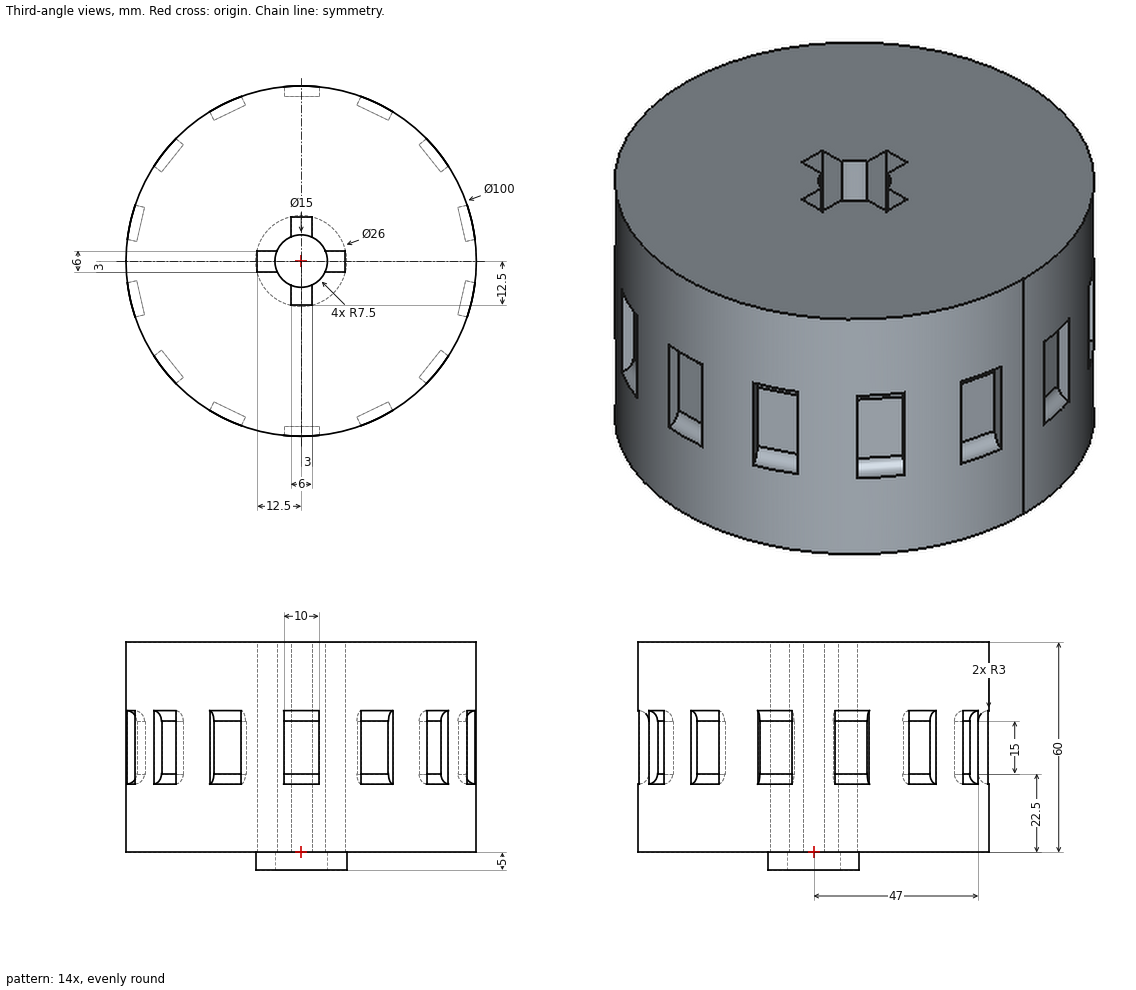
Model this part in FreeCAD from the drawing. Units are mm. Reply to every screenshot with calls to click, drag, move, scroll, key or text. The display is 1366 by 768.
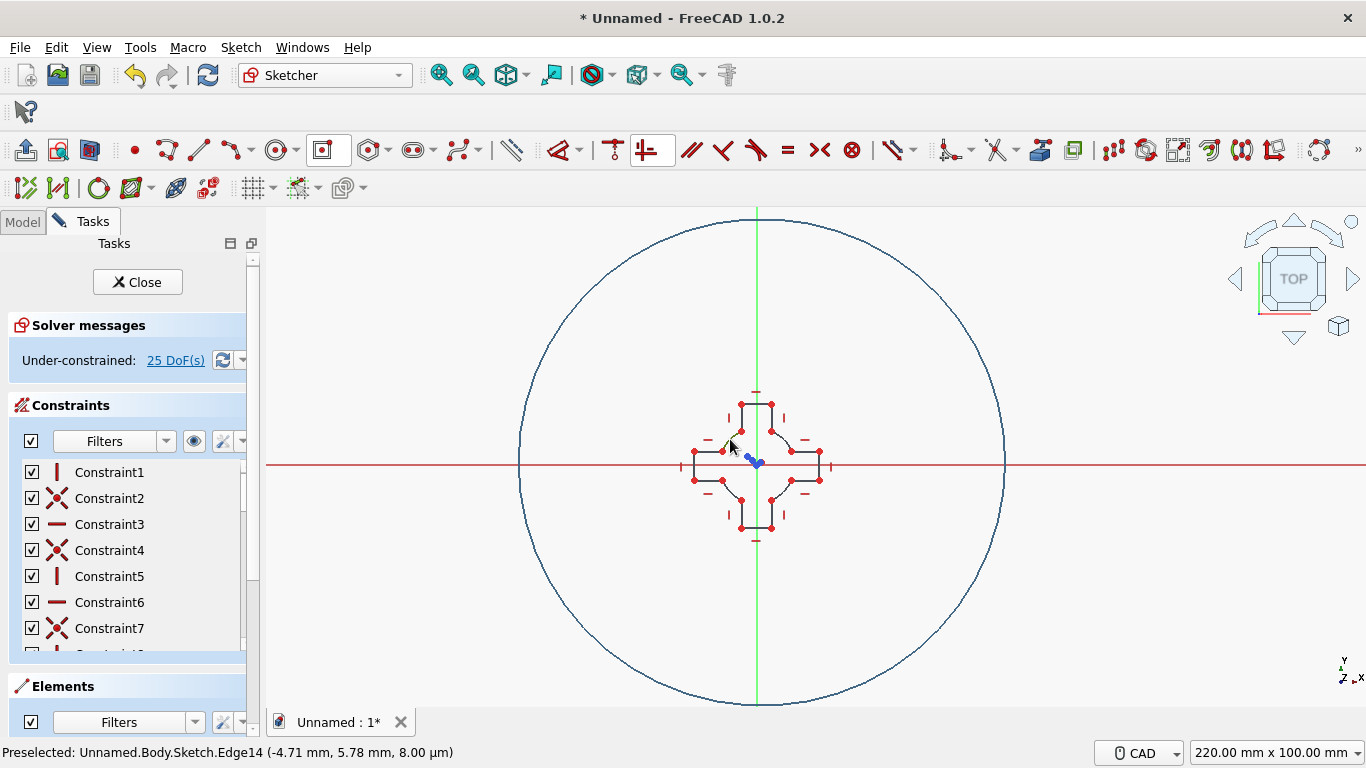
key(c)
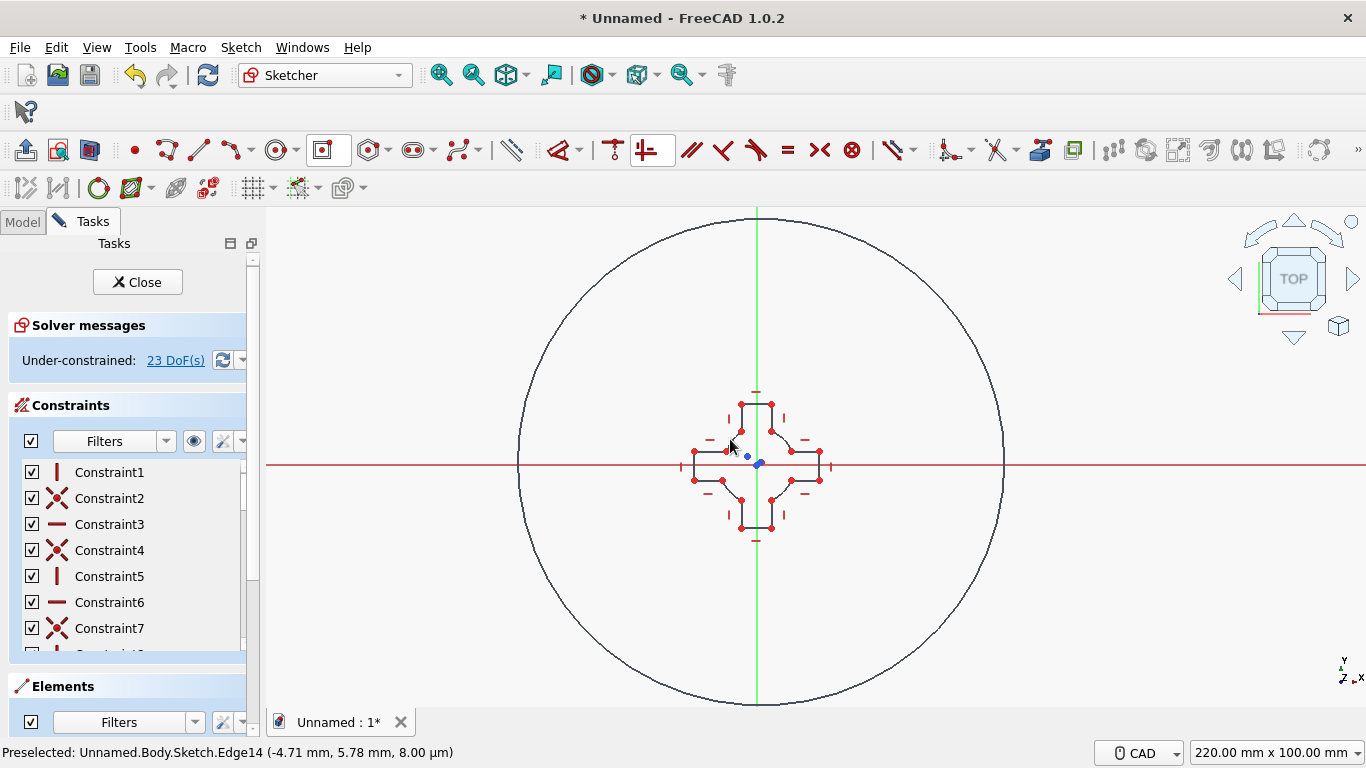
click(933, 290)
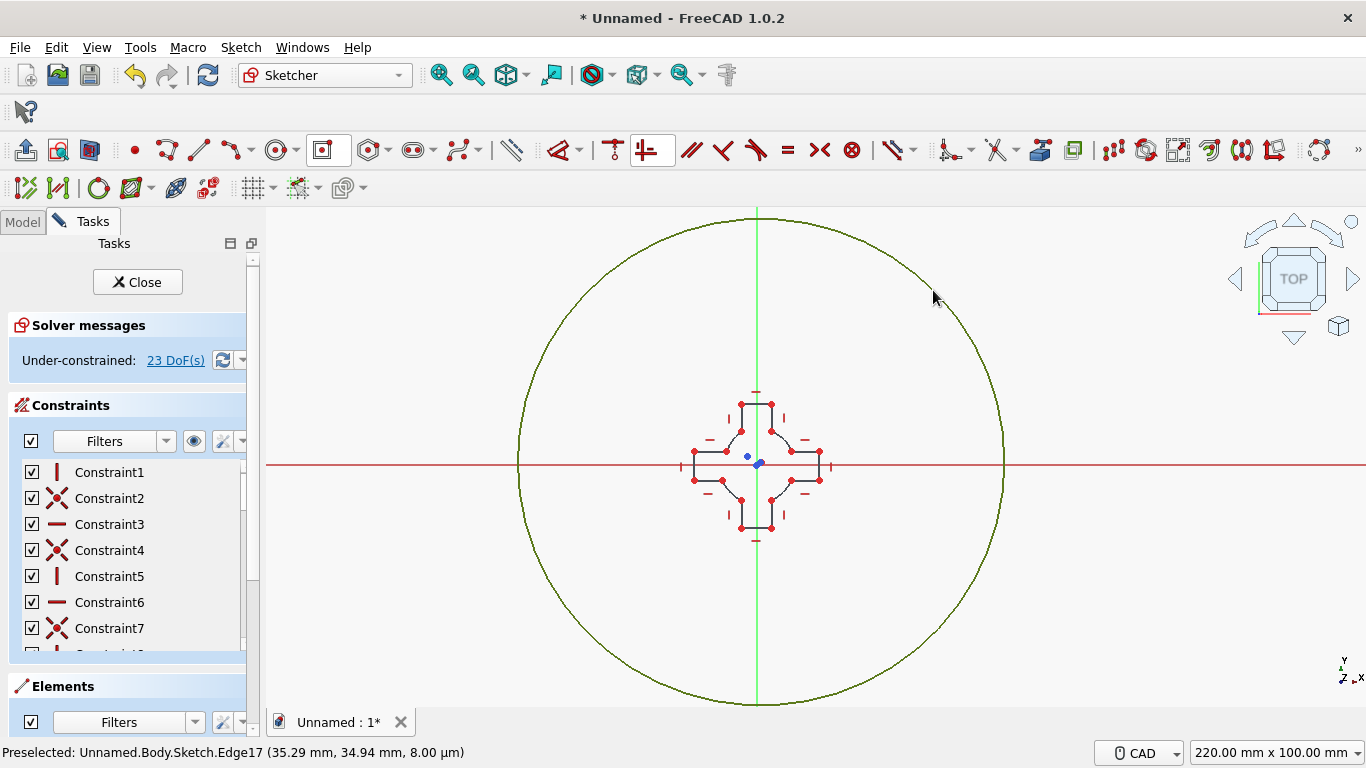
click(784, 440)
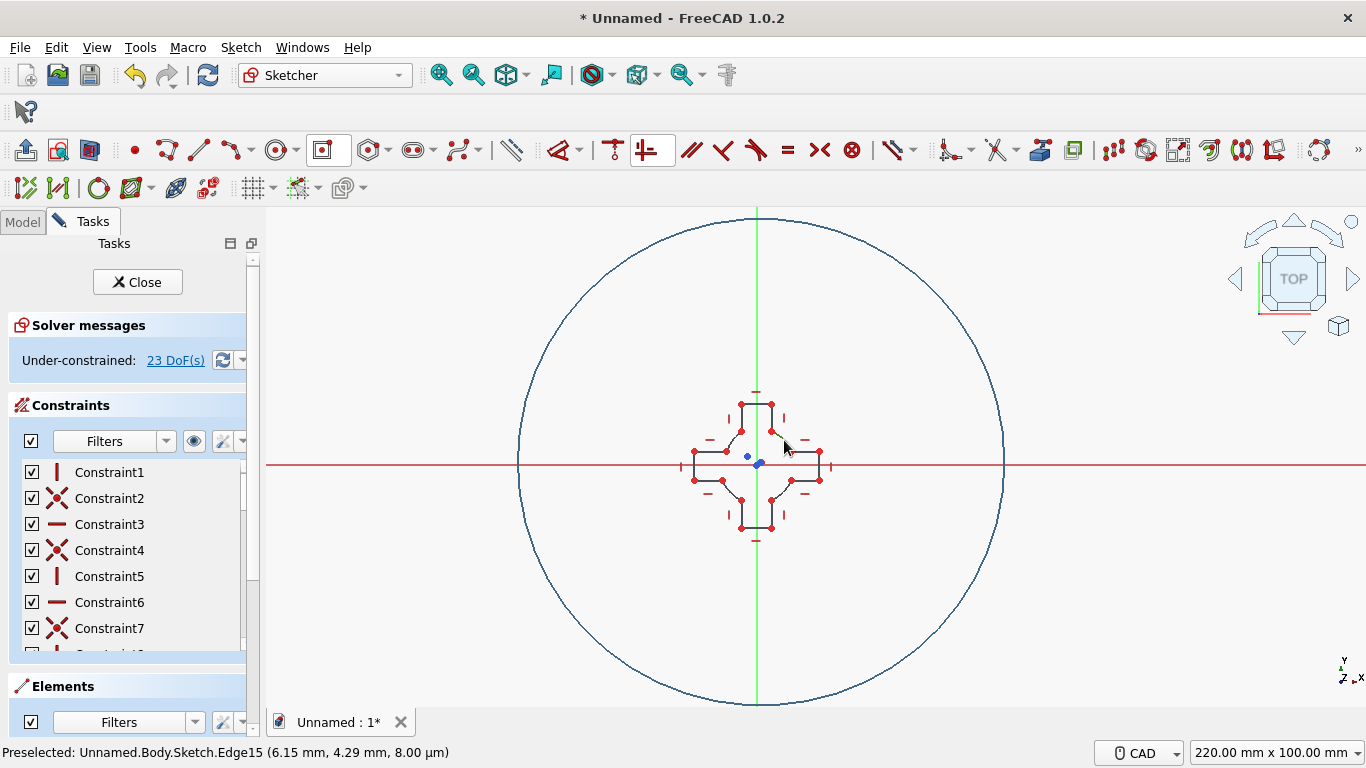
click(614, 150)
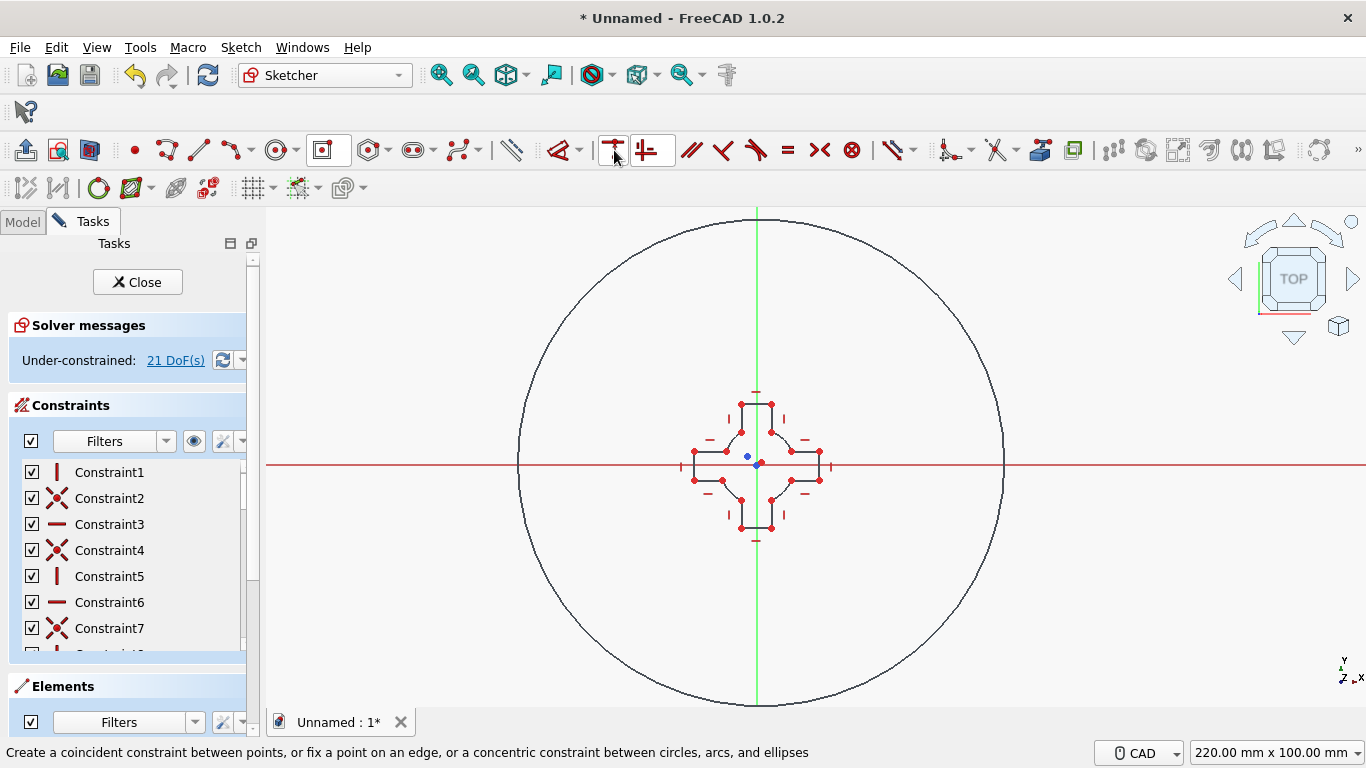
click(933, 290)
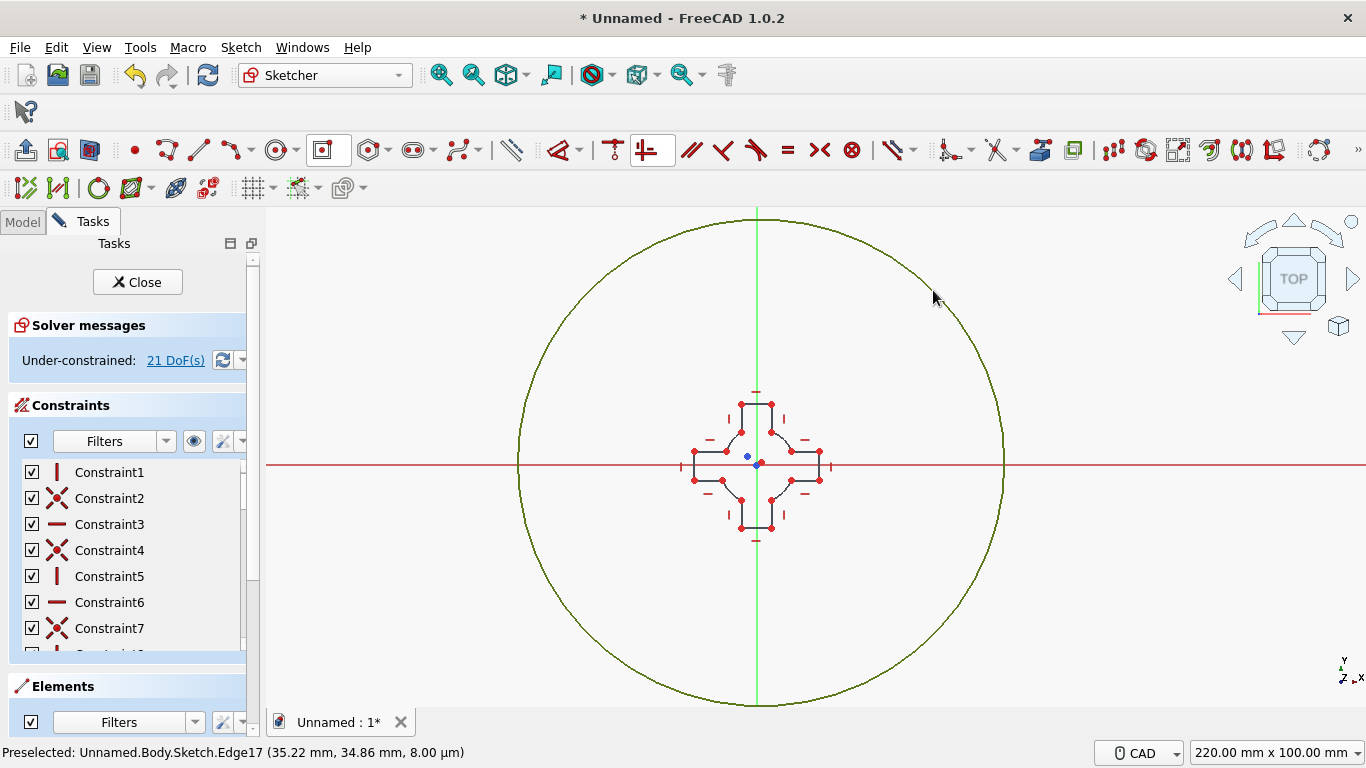
click(783, 492)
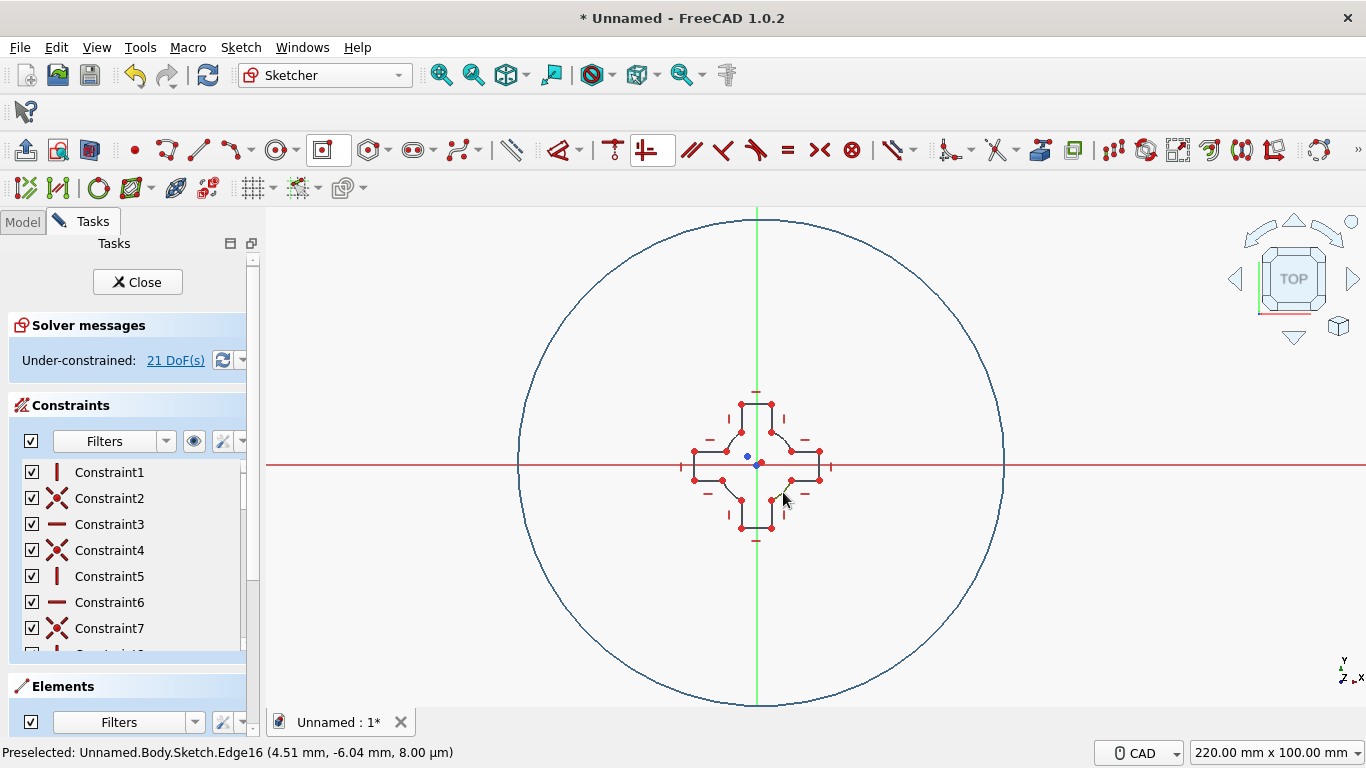
key(c)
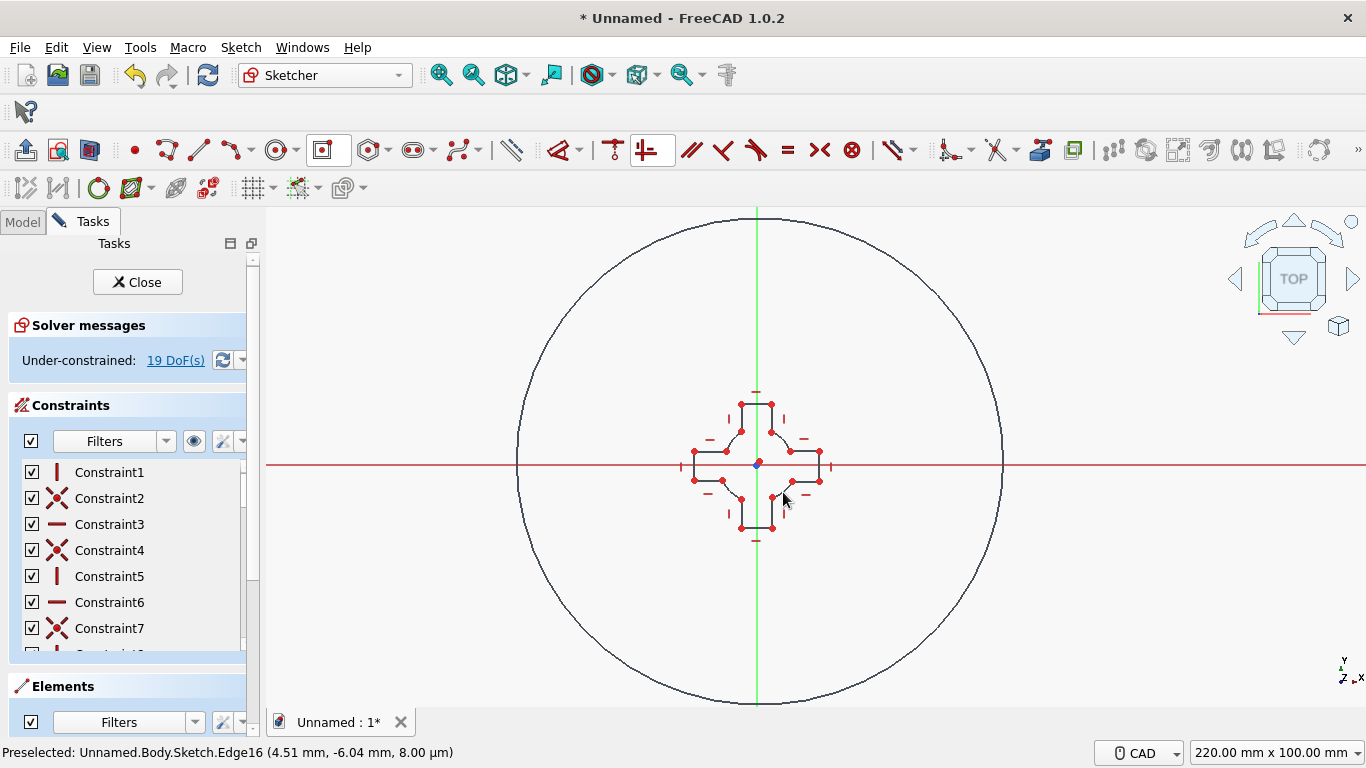
scroll(758, 463, up, 2)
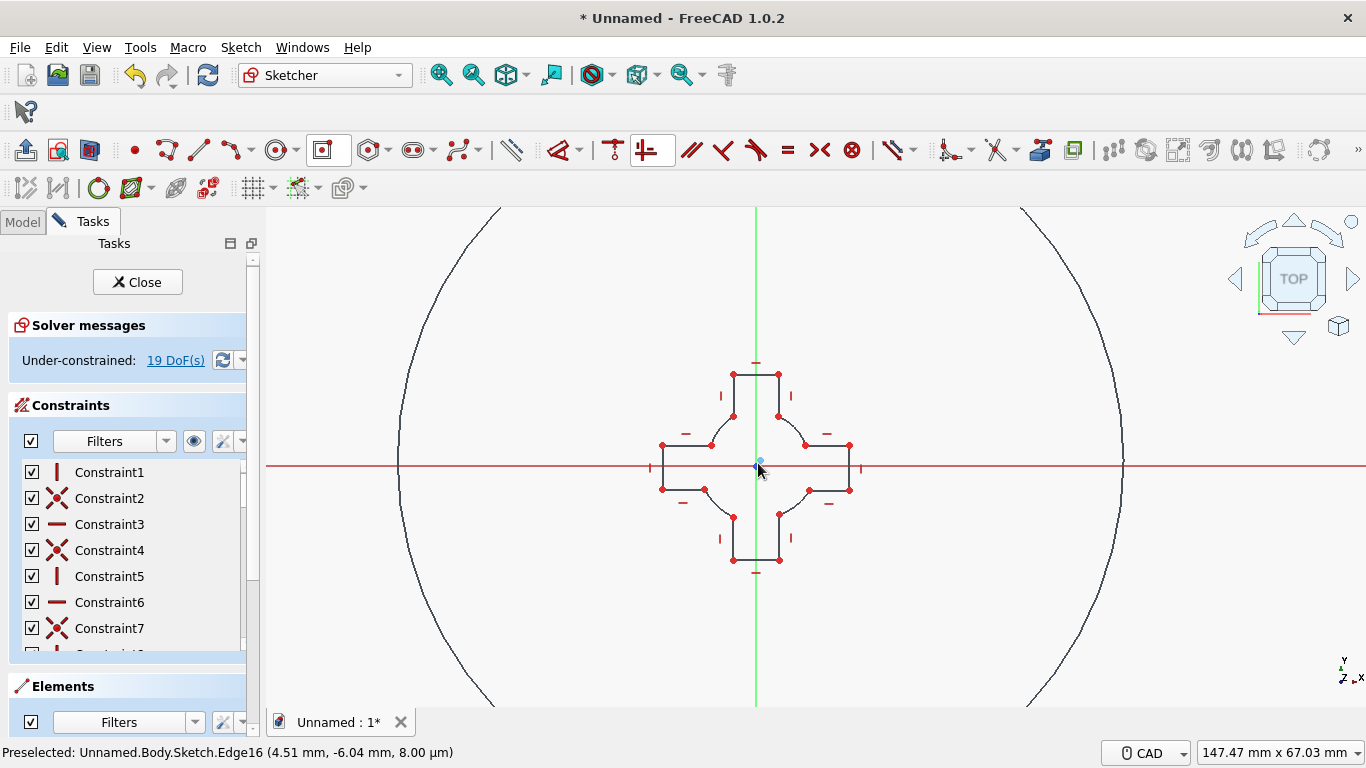
drag(746, 451, 771, 476)